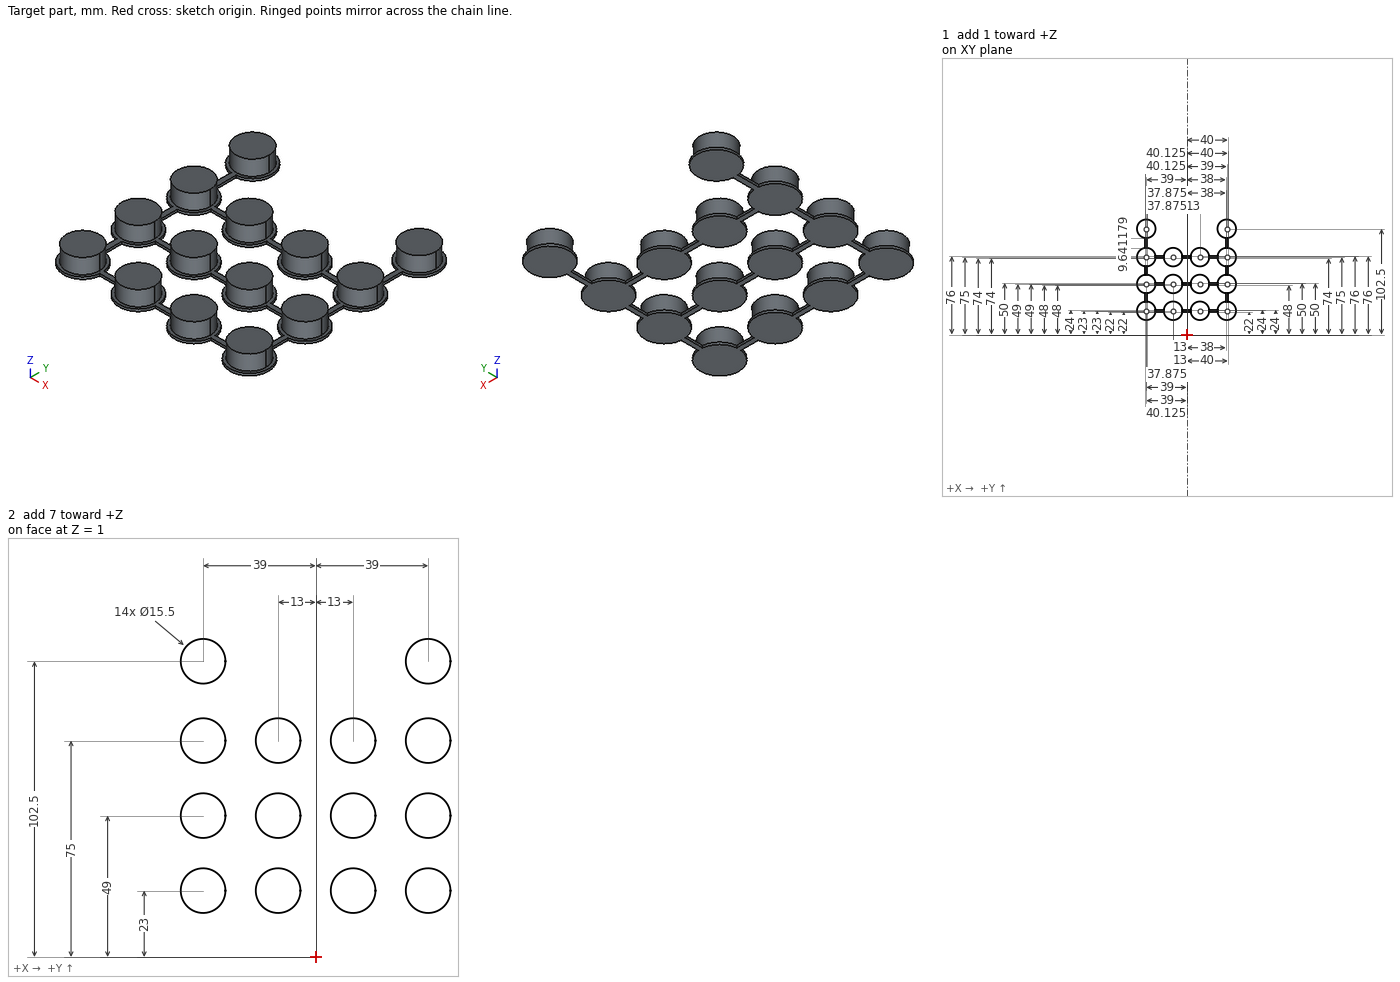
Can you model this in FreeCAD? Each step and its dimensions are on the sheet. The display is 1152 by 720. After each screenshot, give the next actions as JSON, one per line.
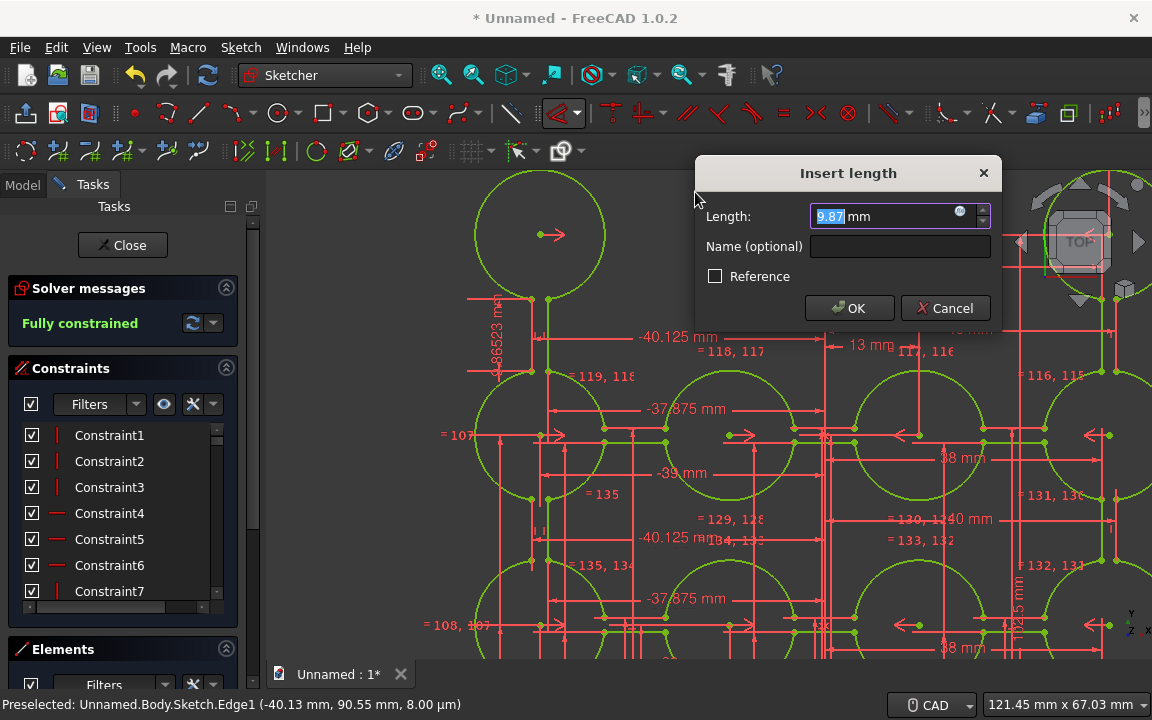
{"action": "type", "text": "9.641179"}
{"action": "key", "text": "Return"}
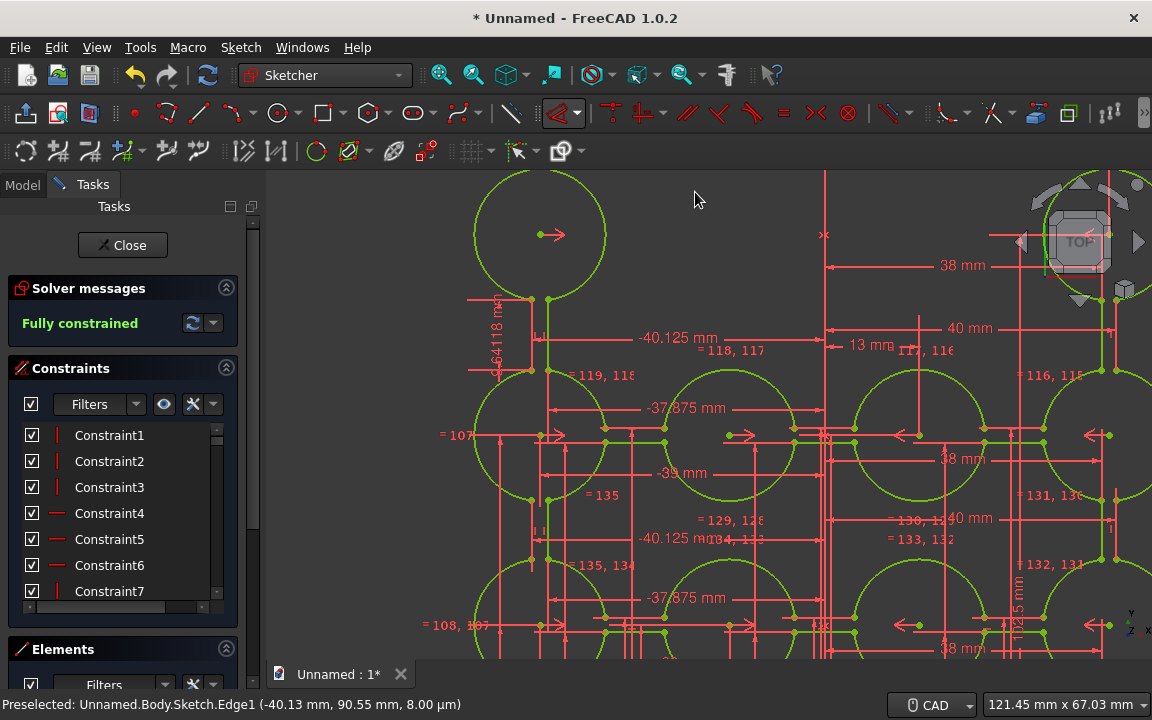
{"action": "left_click", "coordinate": [123, 245]}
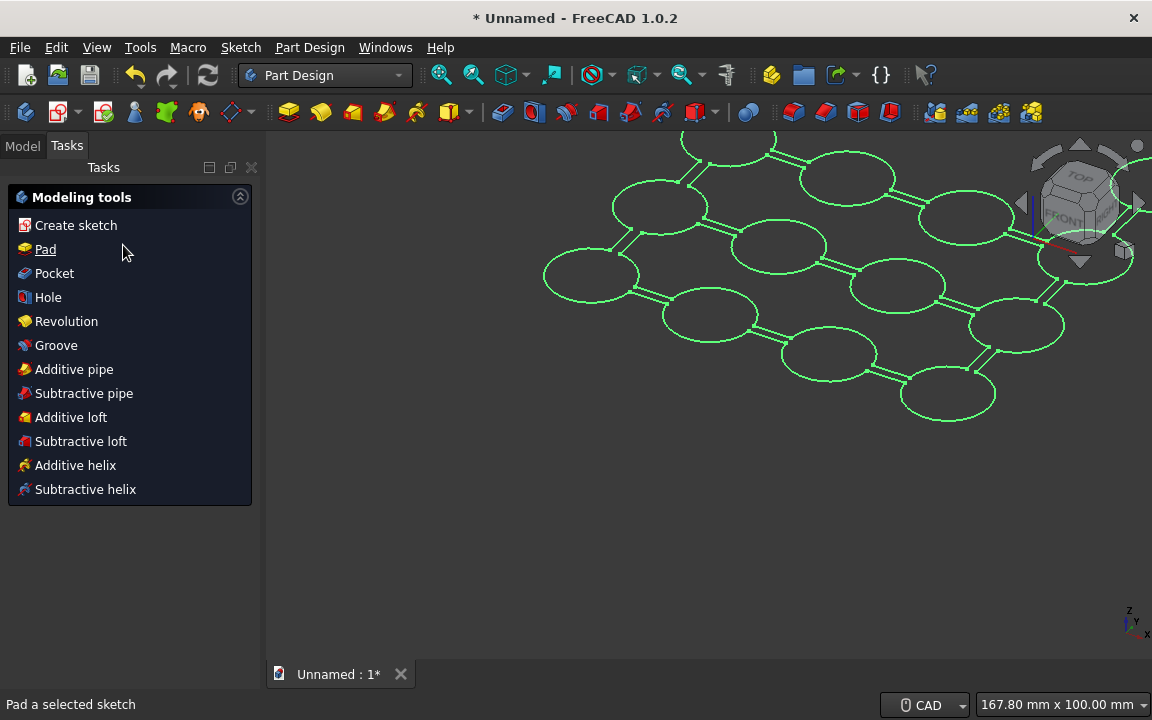
{"action": "left_click", "coordinate": [290, 112]}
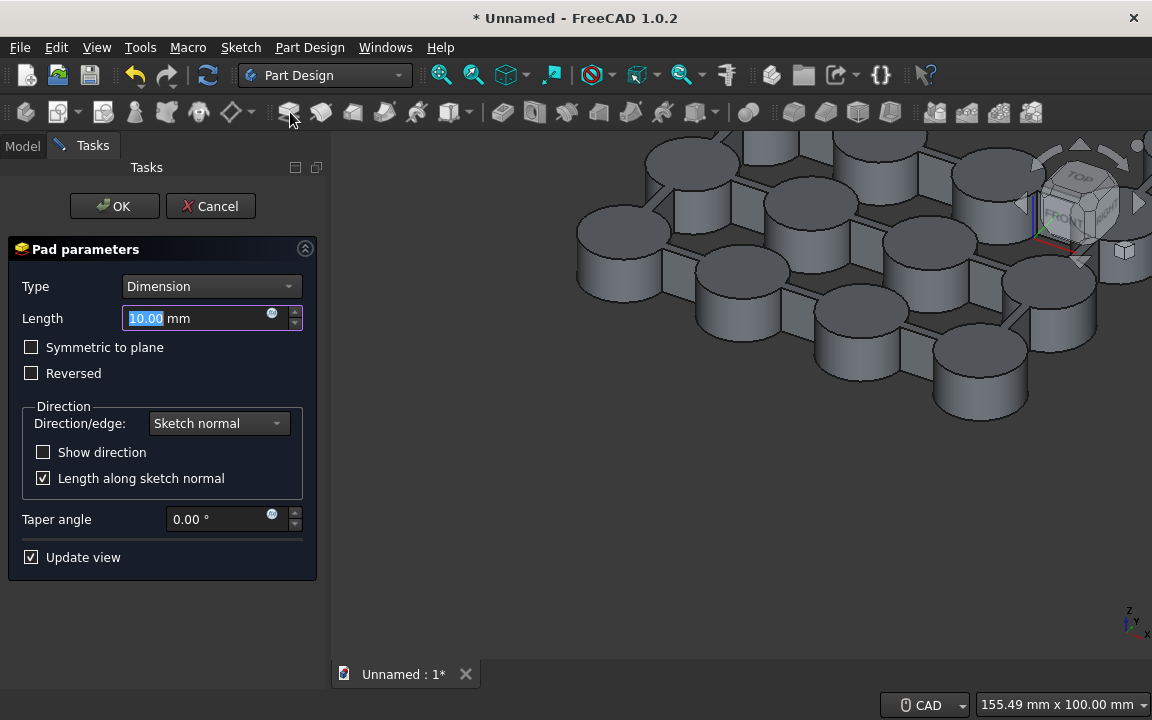
{"action": "type", "text": "1"}
{"action": "key", "text": "Tab"}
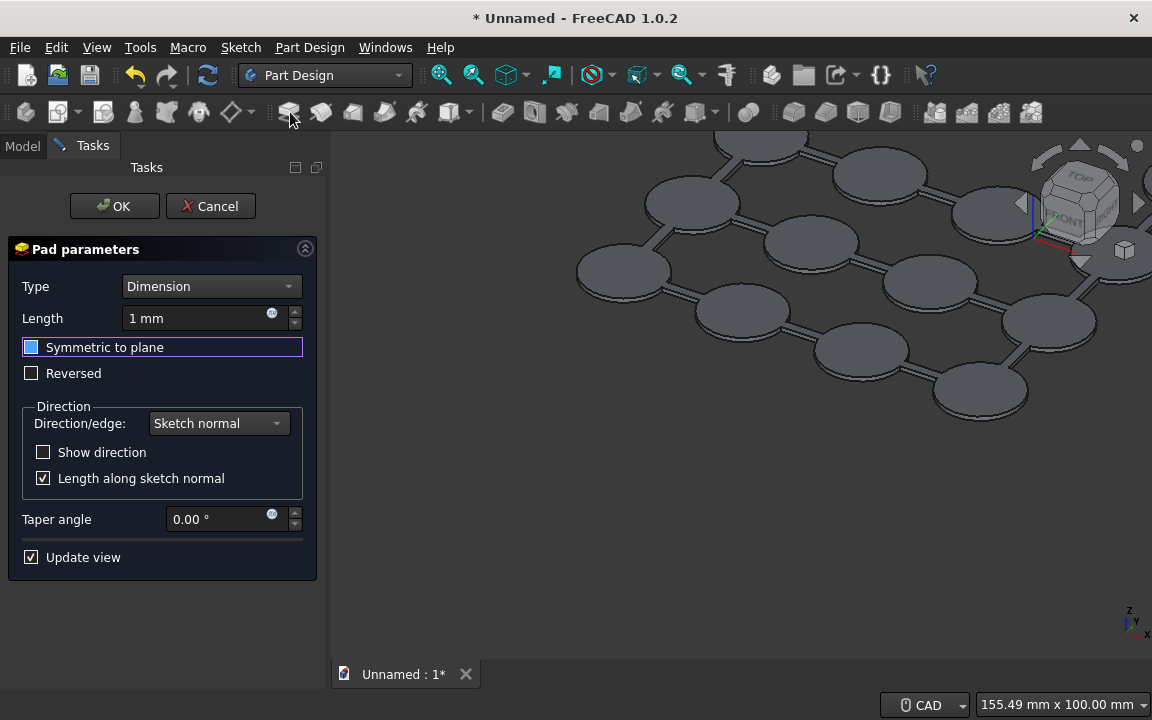
{"action": "left_click", "coordinate": [115, 206]}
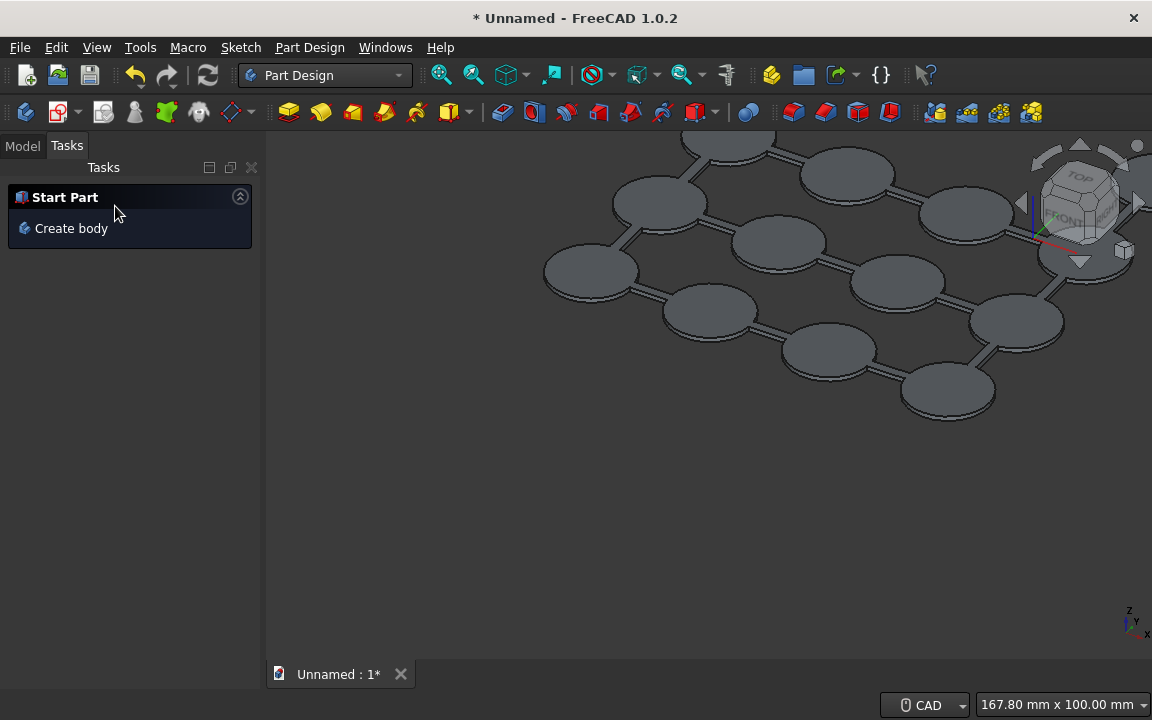
{"action": "left_click", "coordinate": [442, 76]}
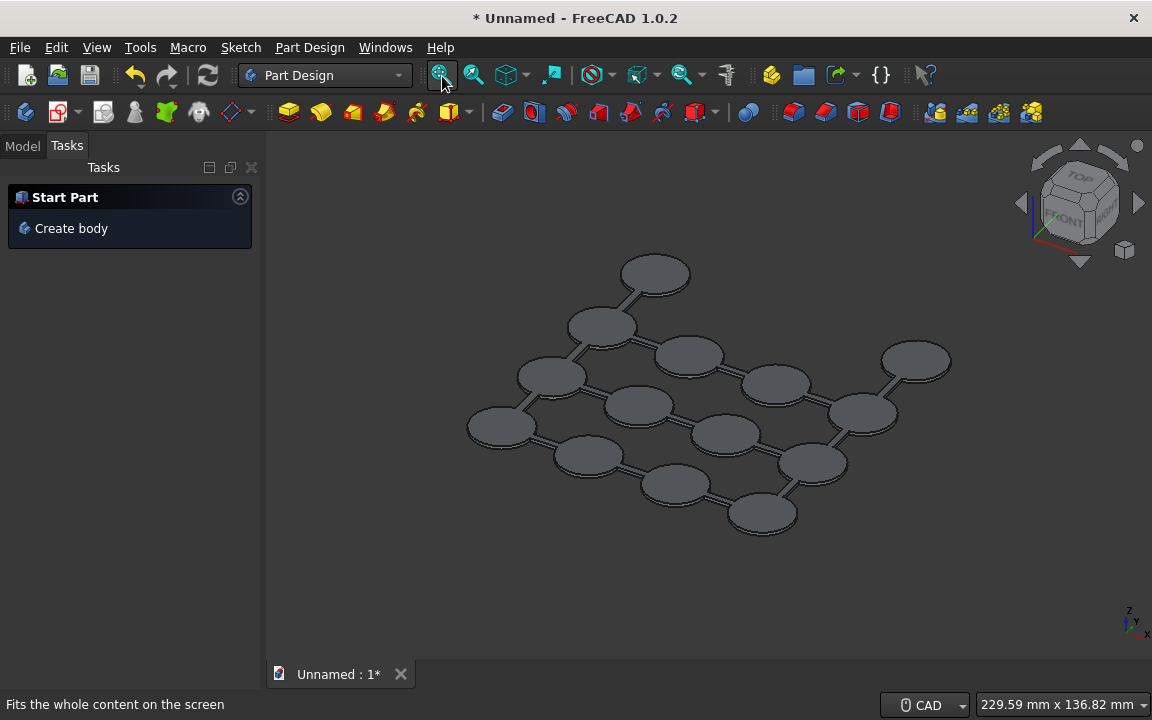
{"action": "left_click", "coordinate": [636, 404]}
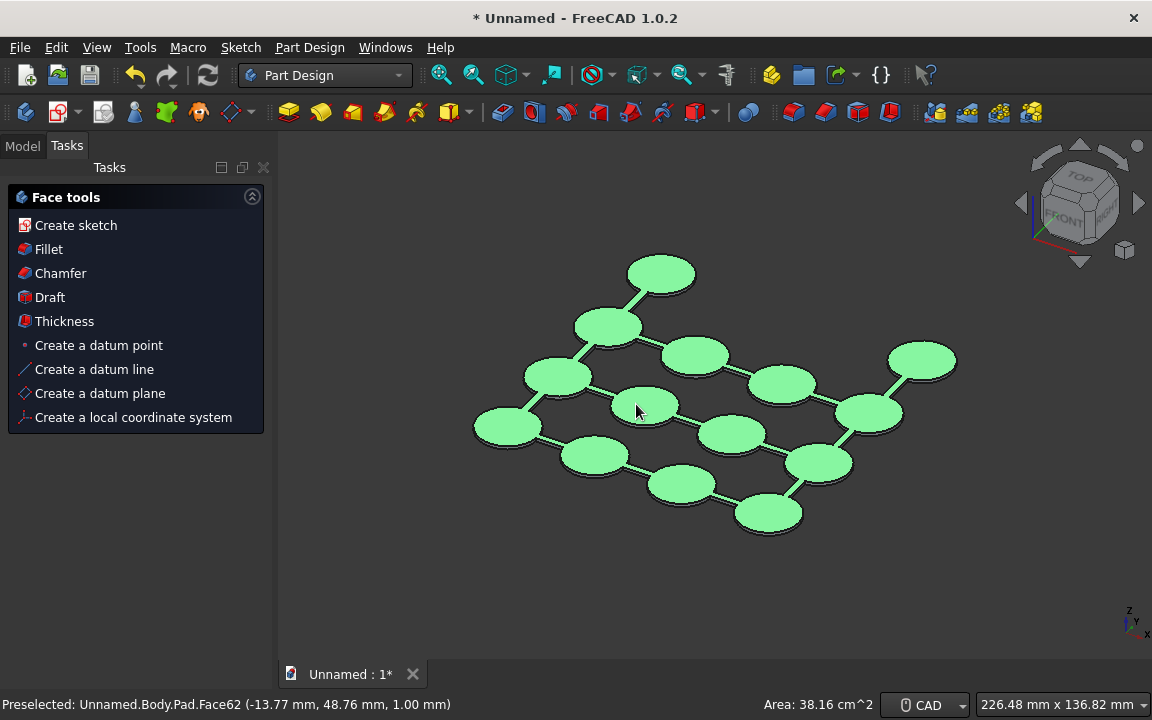
{"action": "left_click", "coordinate": [58, 112]}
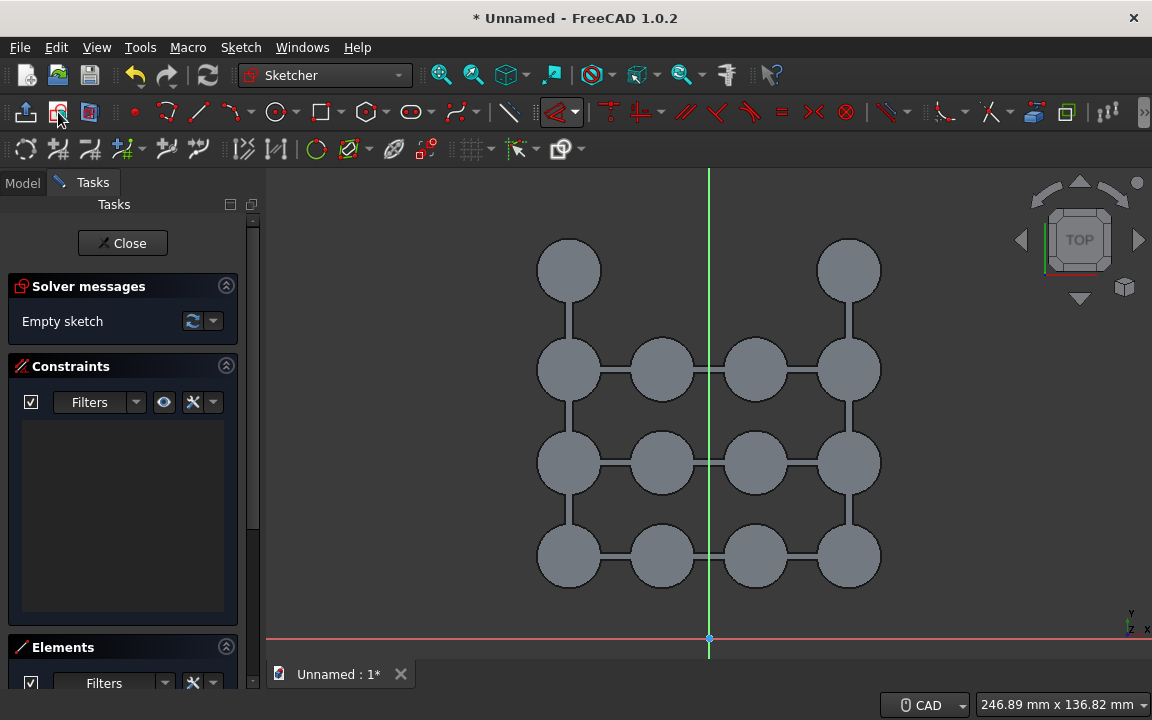
{"action": "scroll", "coordinate": [331, 290], "scroll_direction": "down", "scroll_amount": 1}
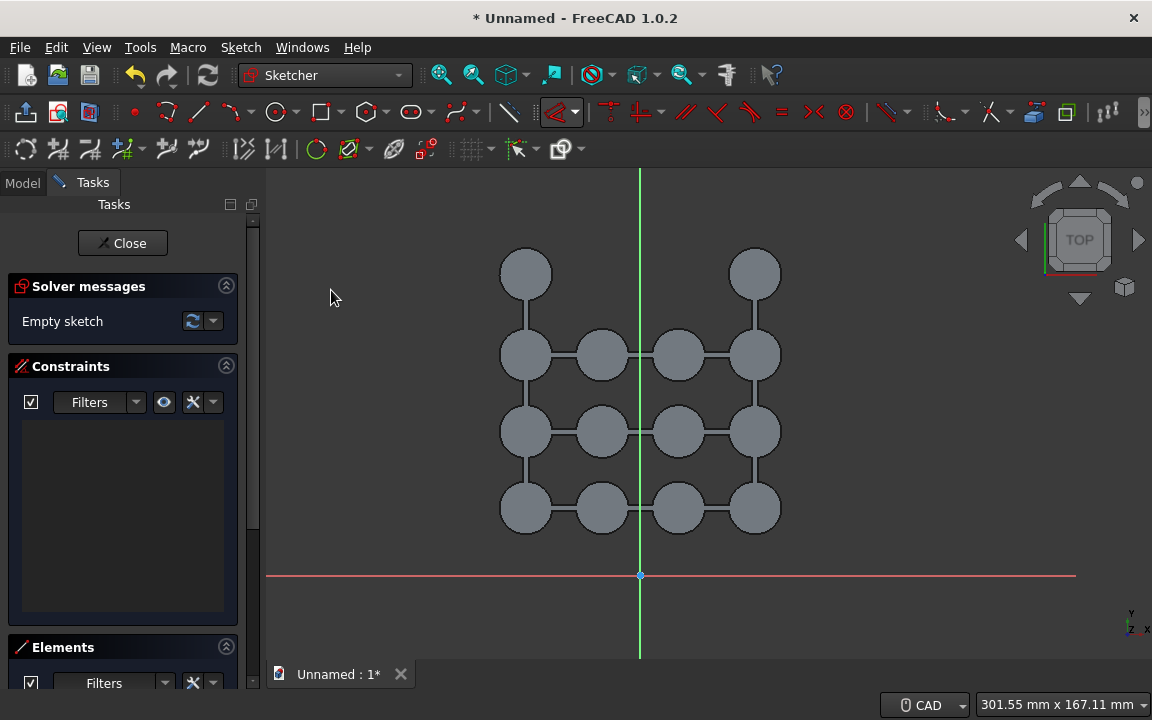
{"action": "left_click", "coordinate": [276, 112]}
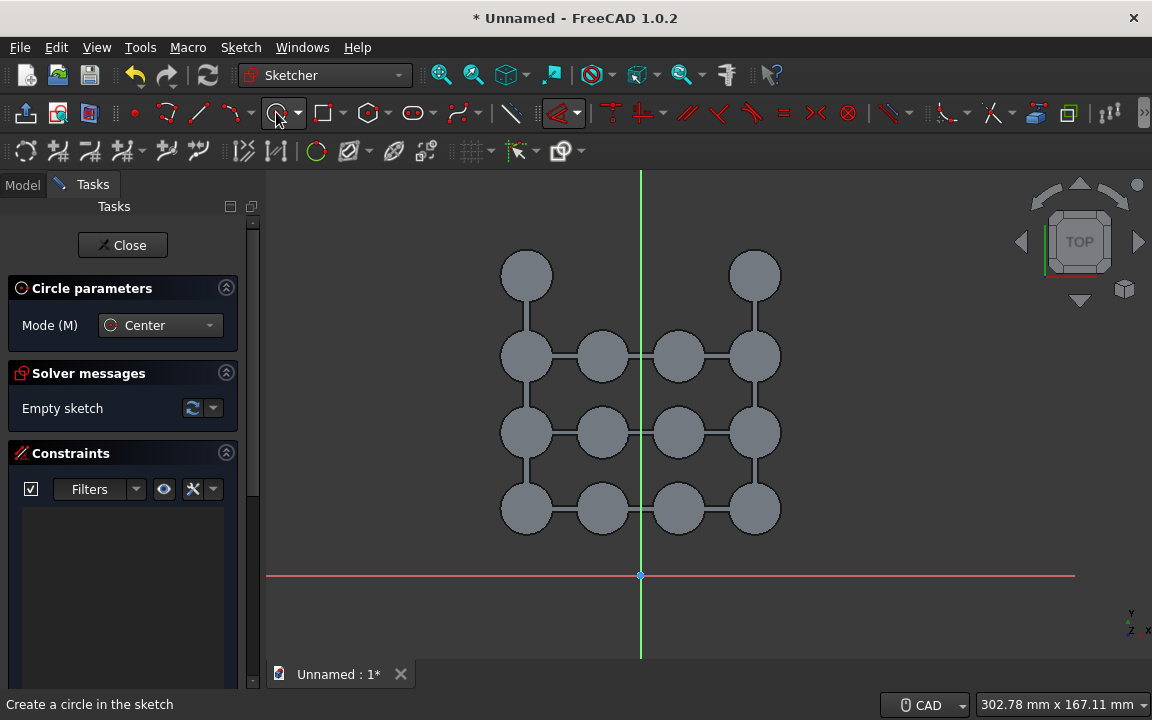
{"action": "left_click", "coordinate": [527, 276]}
{"action": "mouse_move", "coordinate": [543, 260]}